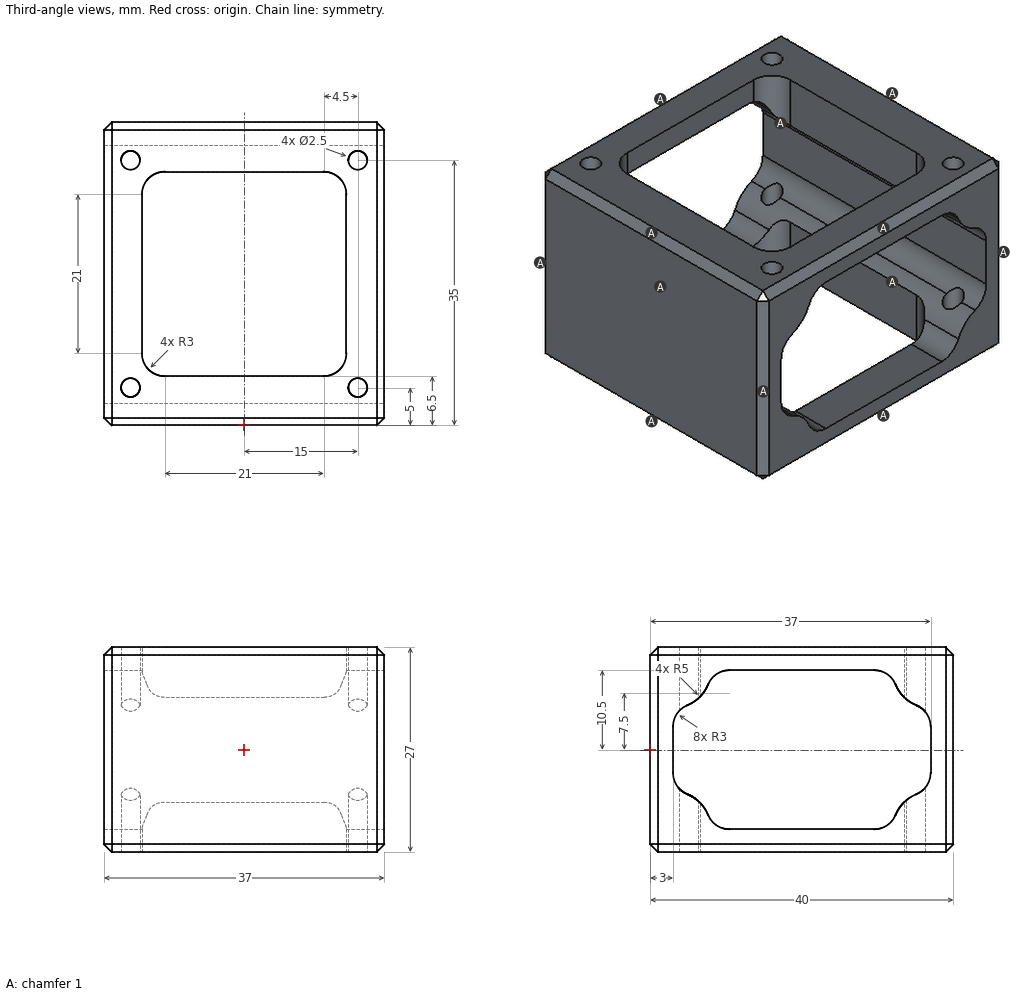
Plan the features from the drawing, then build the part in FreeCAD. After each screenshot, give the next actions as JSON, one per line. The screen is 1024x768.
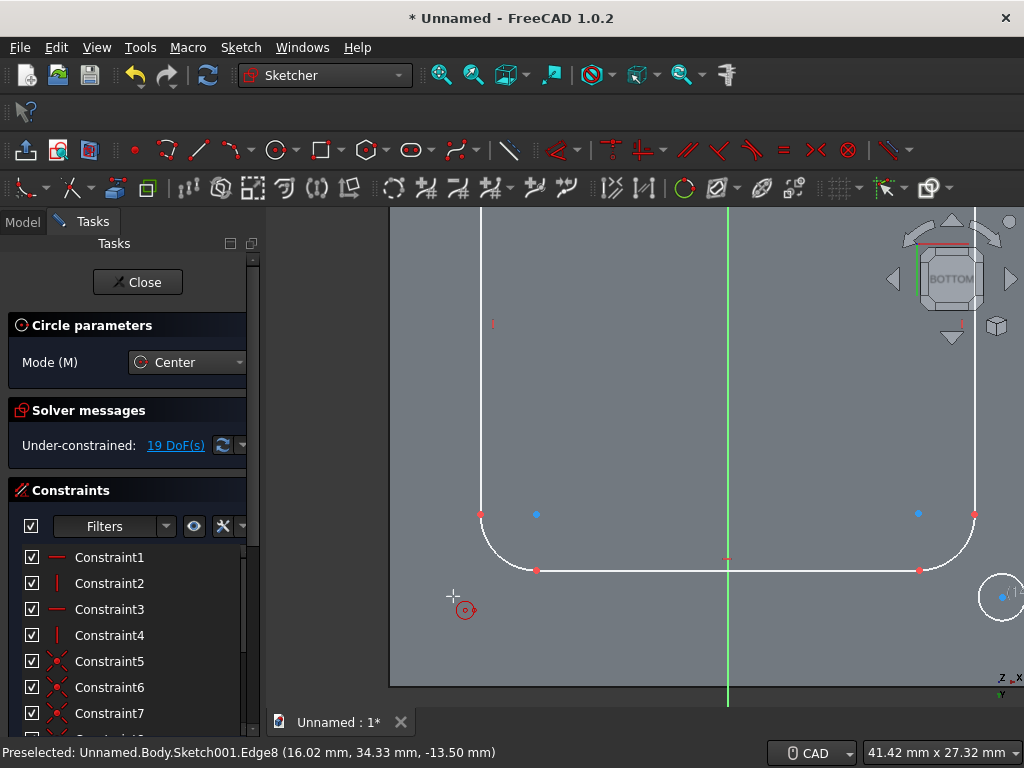
{"action": "left_click", "coordinate": [453, 596]}
{"action": "left_click", "coordinate": [470, 580]}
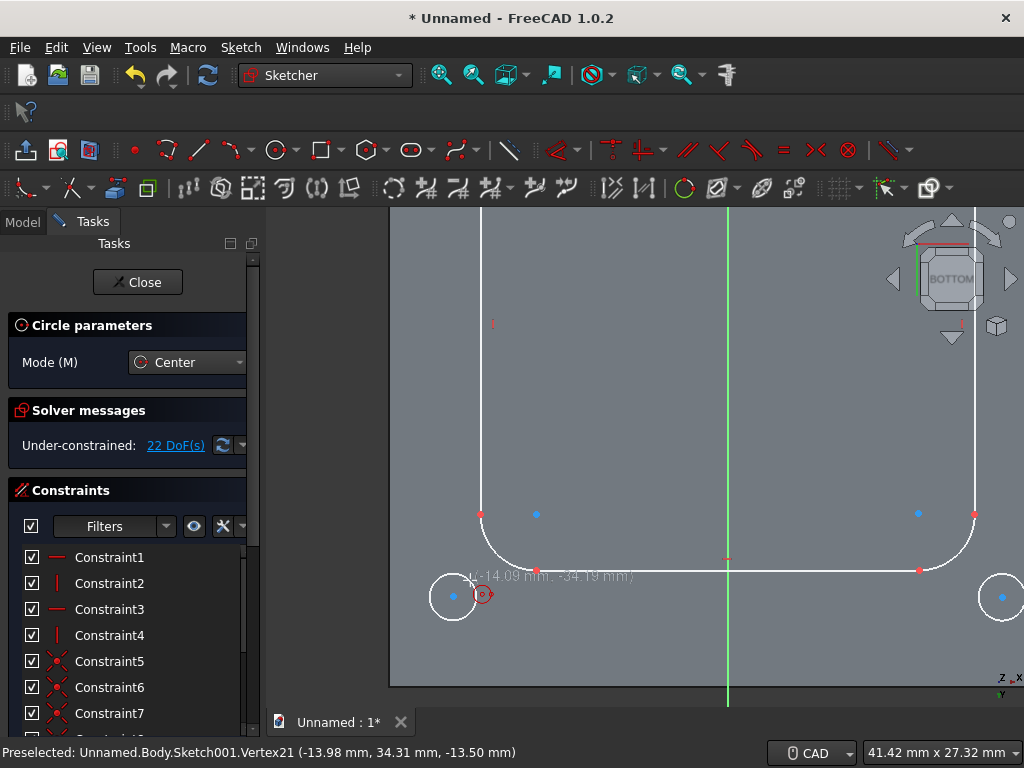
{"action": "scroll", "coordinate": [453, 596], "scroll_direction": "down", "scroll_amount": 4}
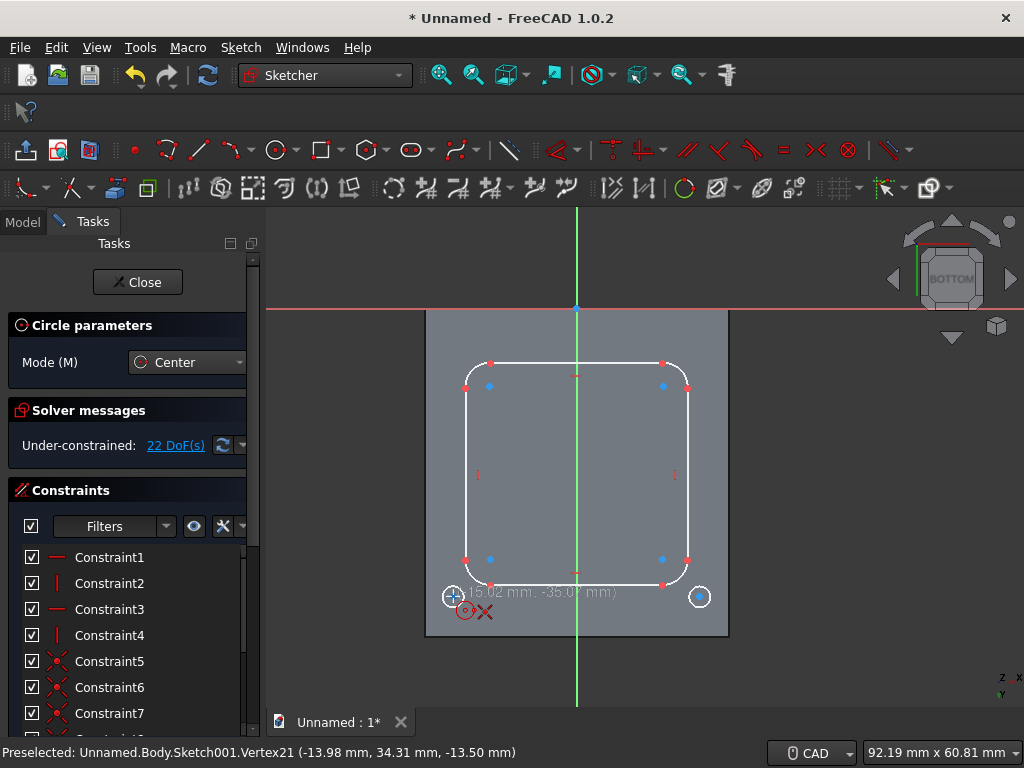
{"action": "scroll", "coordinate": [700, 350], "scroll_direction": "up", "scroll_amount": 4}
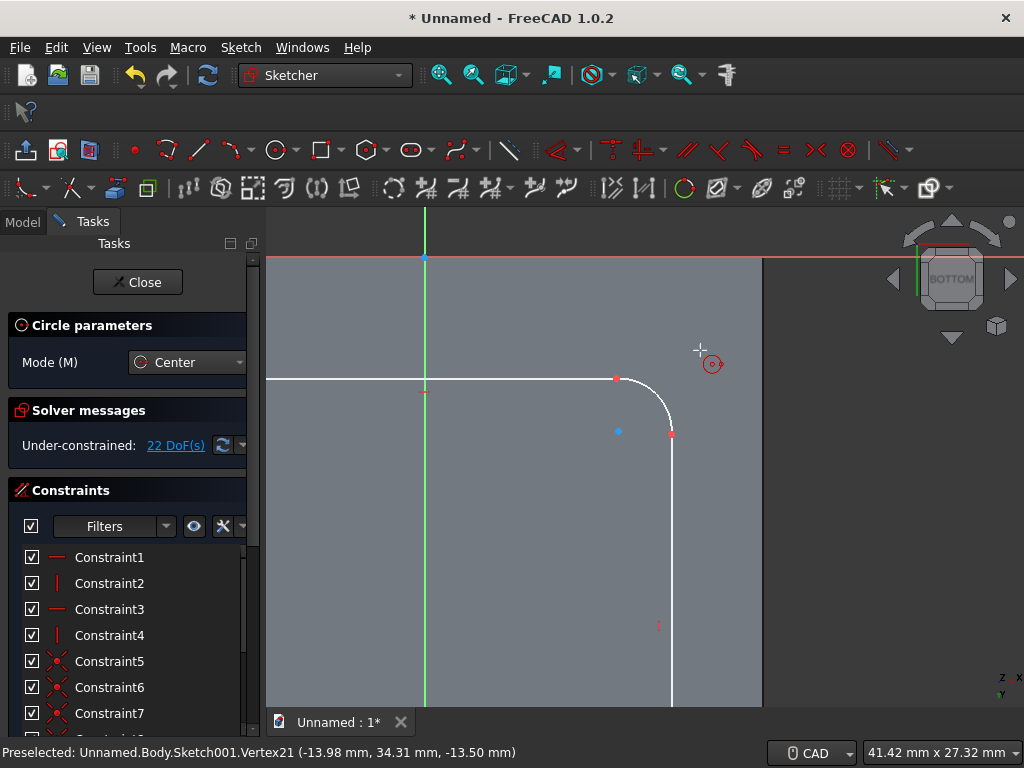
{"action": "left_click", "coordinate": [699, 349]}
{"action": "left_click", "coordinate": [715, 333]}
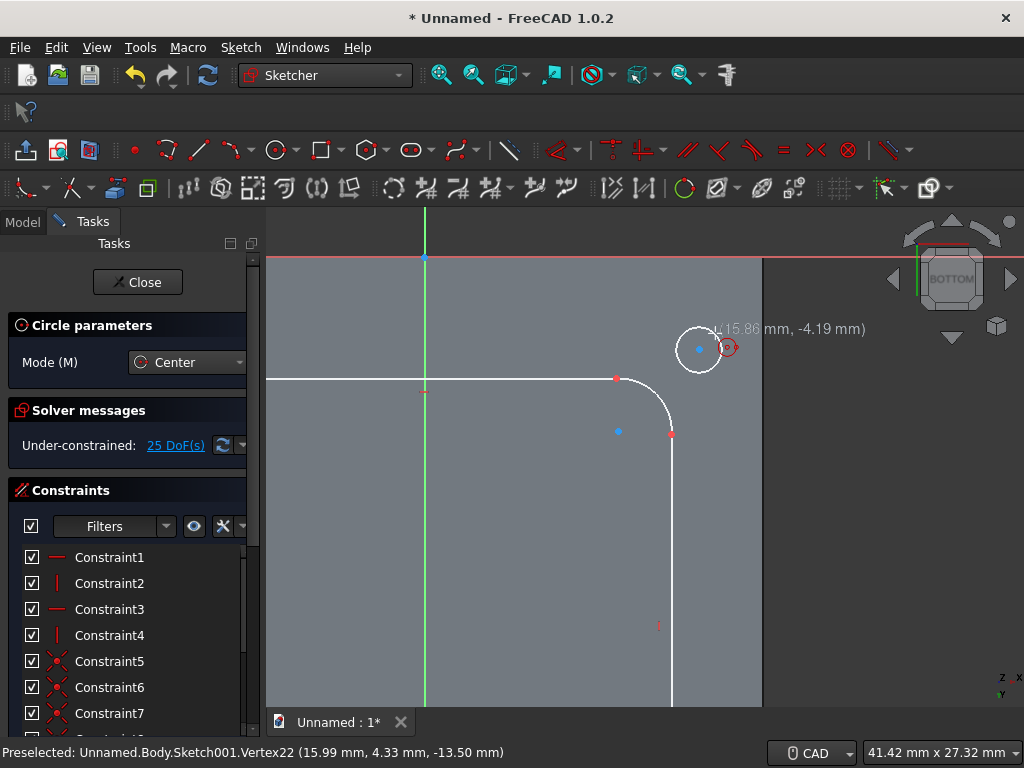
{"action": "scroll", "coordinate": [700, 349], "scroll_direction": "down", "scroll_amount": 4}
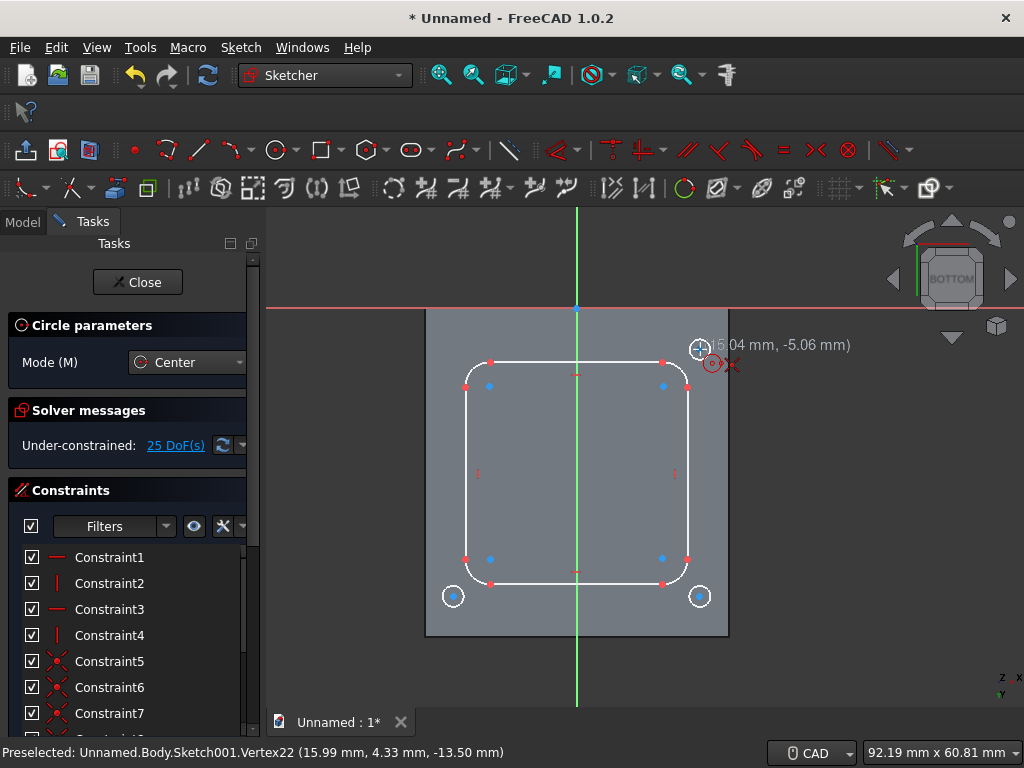
{"action": "scroll", "coordinate": [453, 349], "scroll_direction": "up", "scroll_amount": 4}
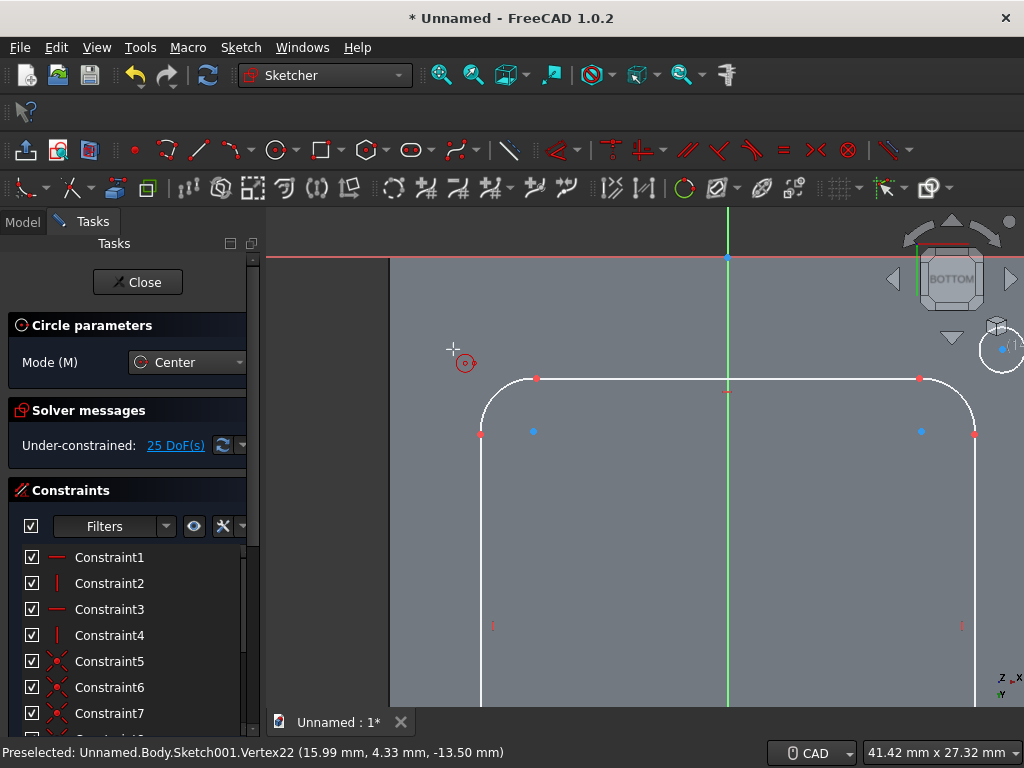
{"action": "left_click", "coordinate": [453, 349]}
{"action": "left_click", "coordinate": [470, 333]}
{"action": "key", "text": "Escape"}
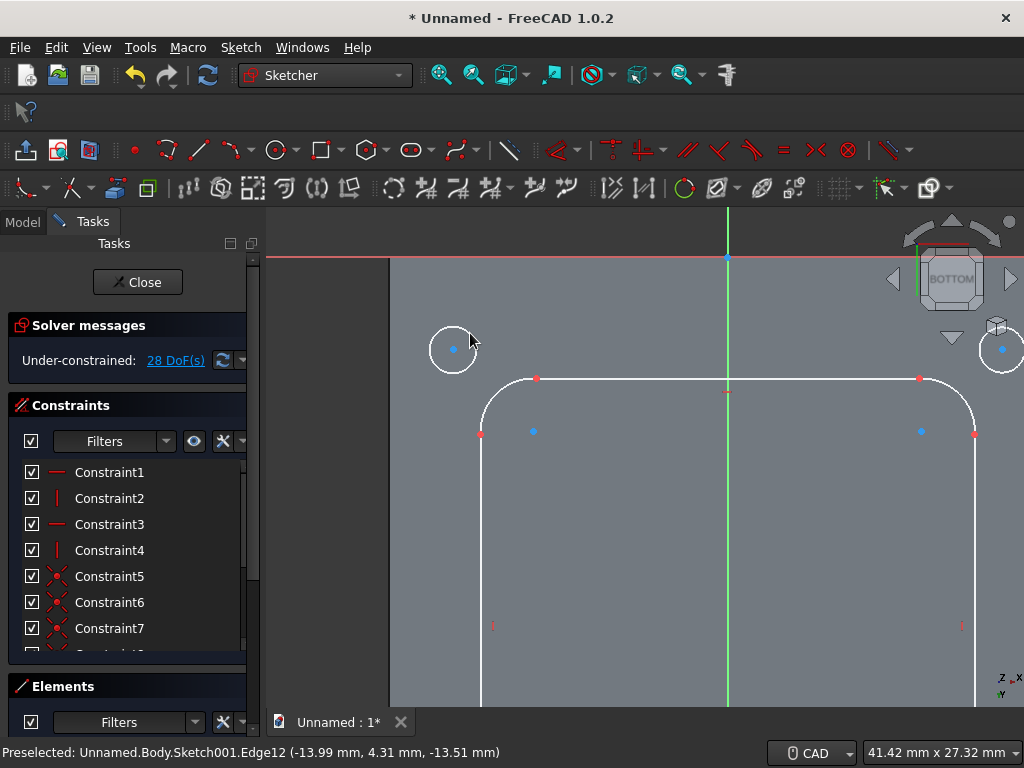
{"action": "left_click", "coordinate": [804, 379]}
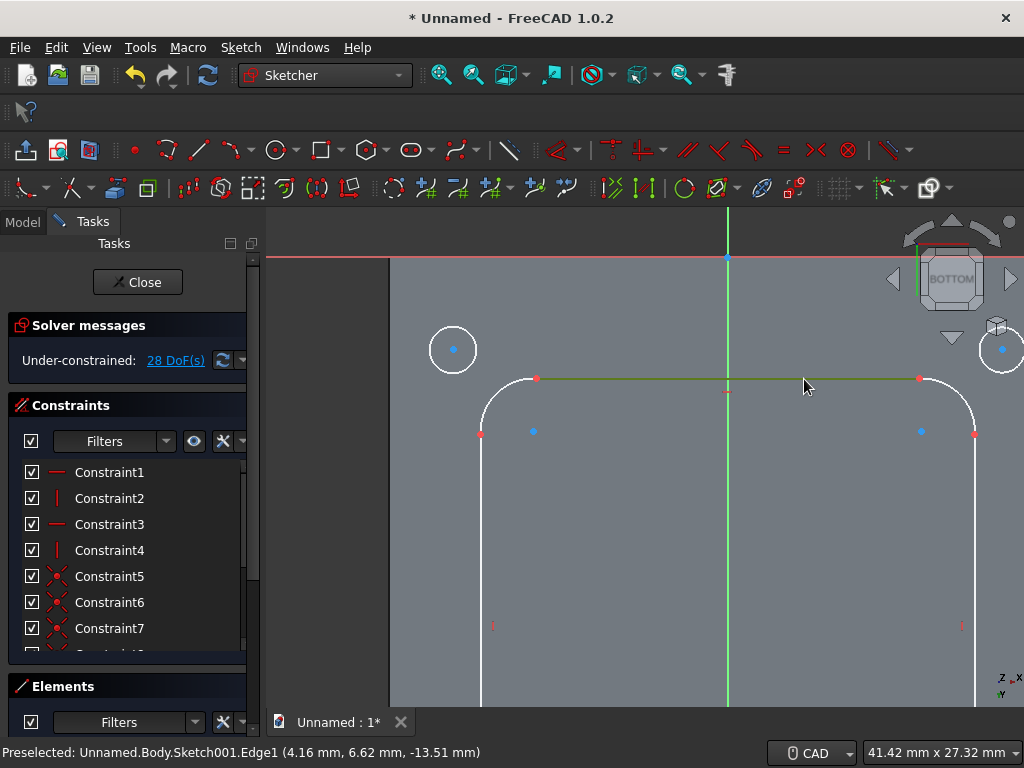
{"action": "left_click", "coordinate": [511, 384]}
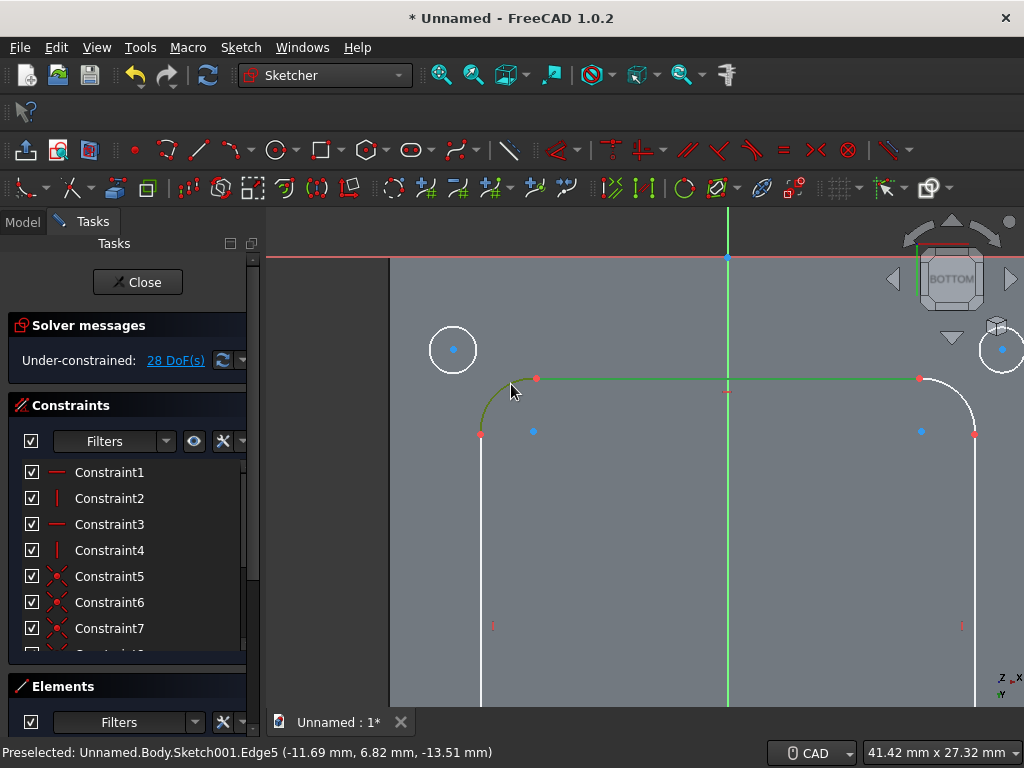
{"action": "key", "text": "t"}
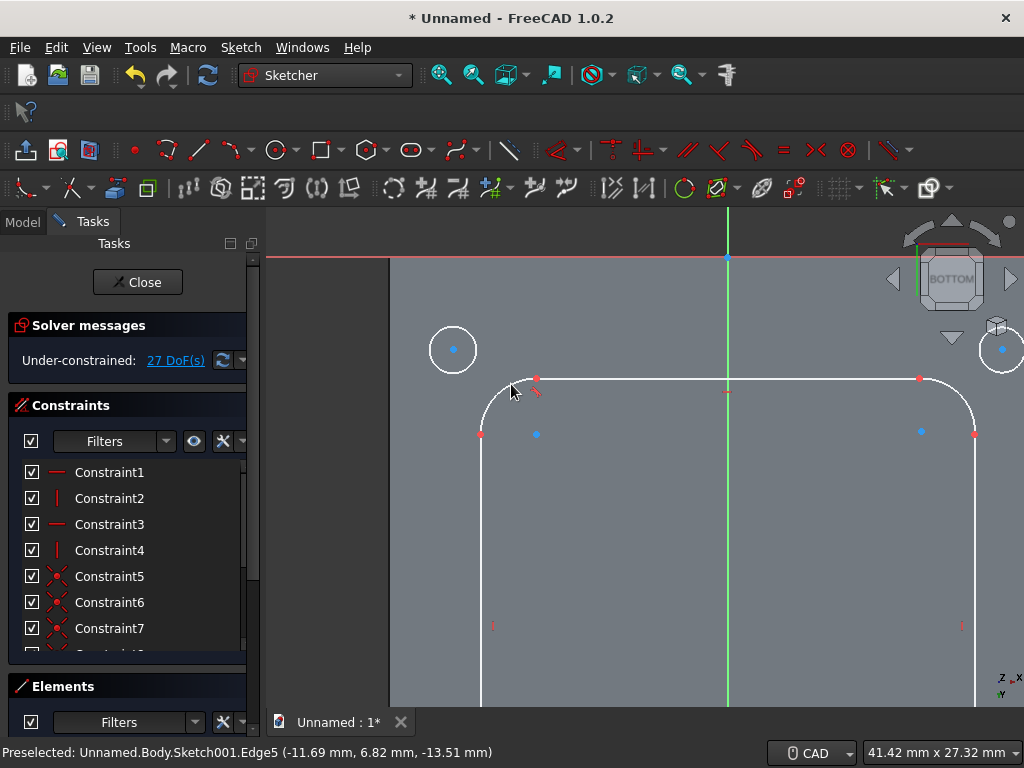
{"action": "left_click", "coordinate": [804, 379]}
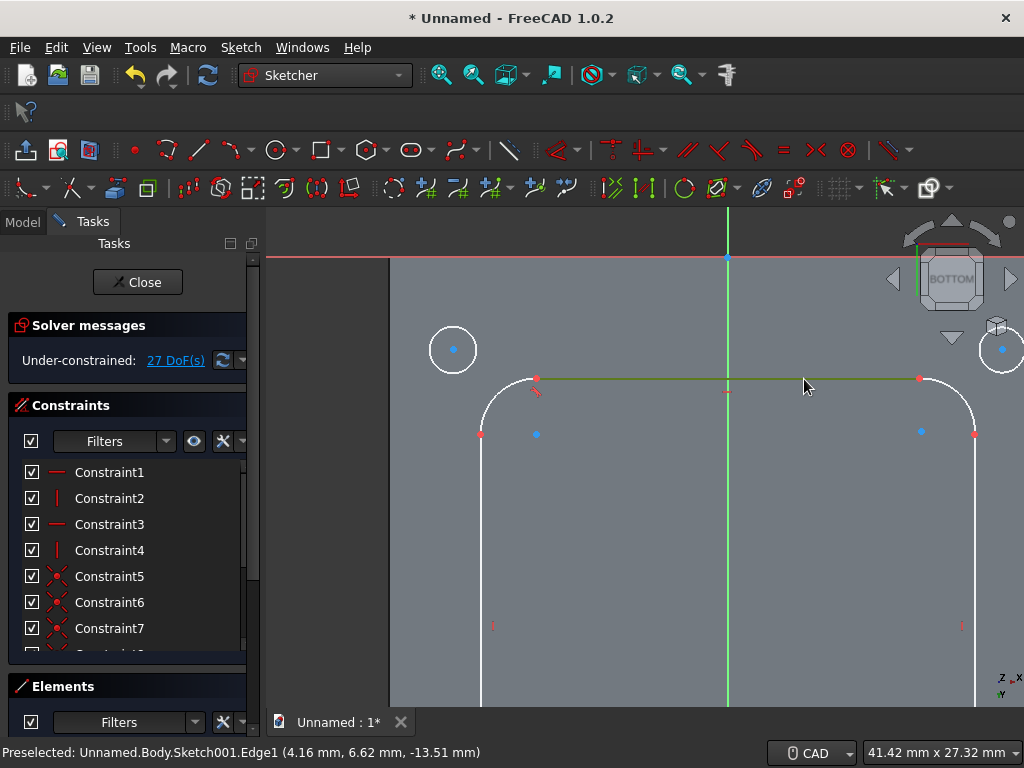
{"action": "scroll", "coordinate": [453, 349], "scroll_direction": "down", "scroll_amount": 4}